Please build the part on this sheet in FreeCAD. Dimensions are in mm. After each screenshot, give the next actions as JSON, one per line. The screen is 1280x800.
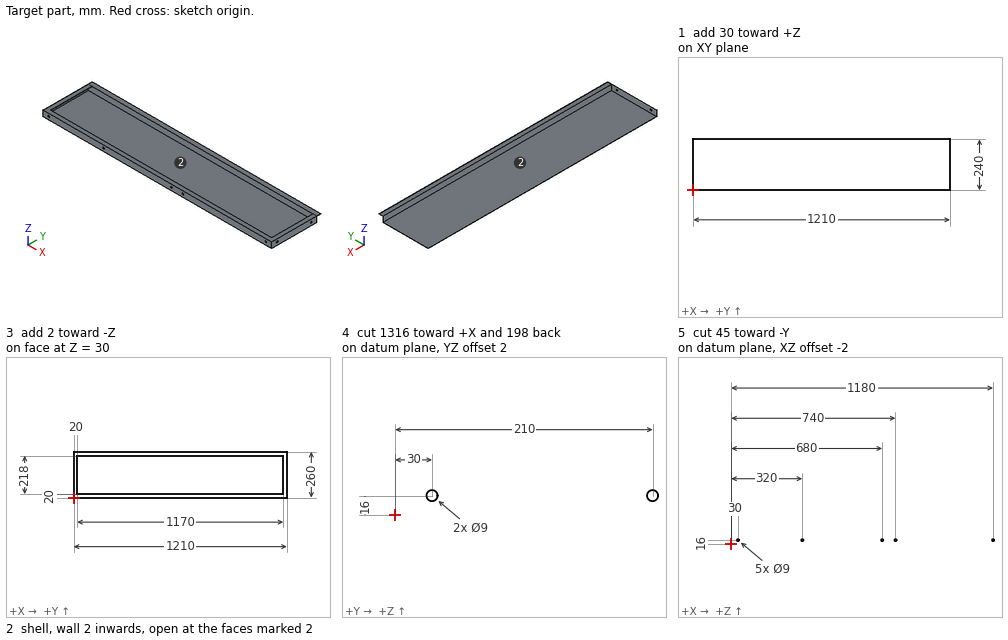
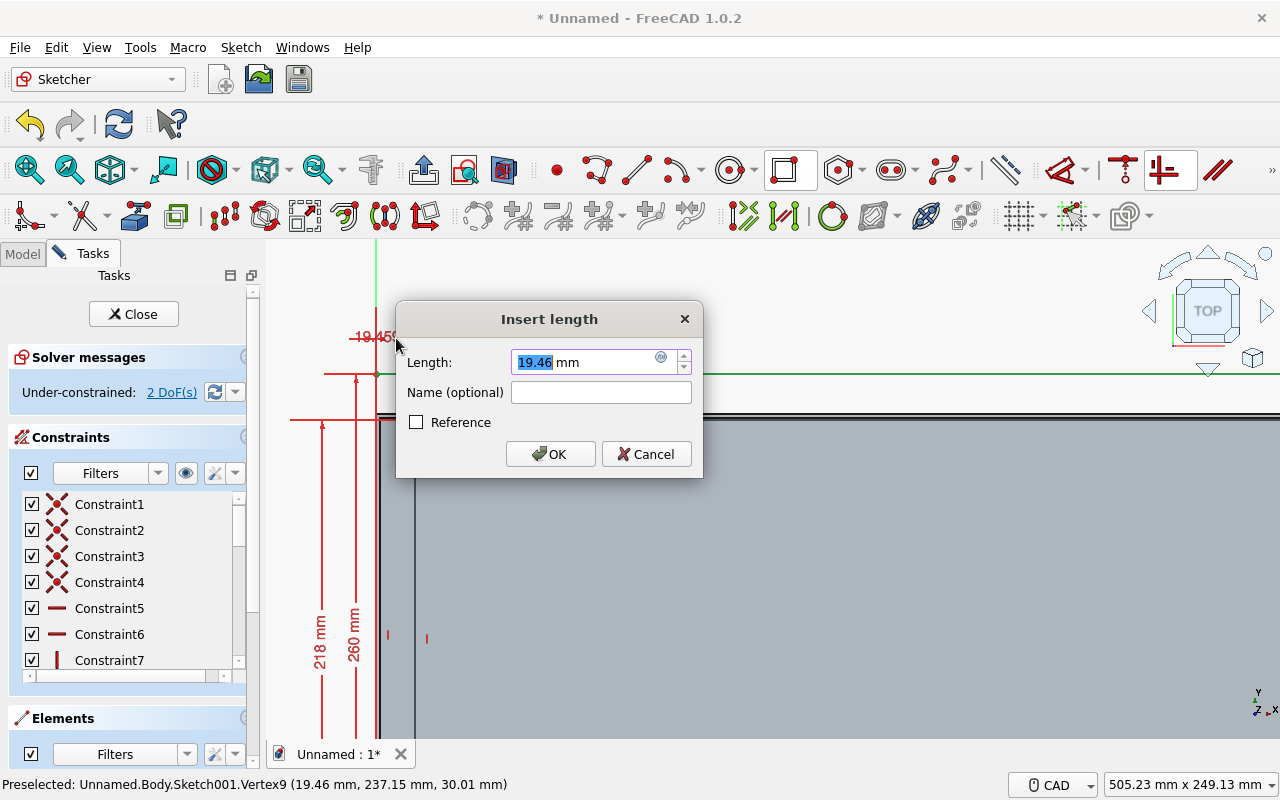
{"action": "type", "text": "20"}
{"action": "key", "text": "Return"}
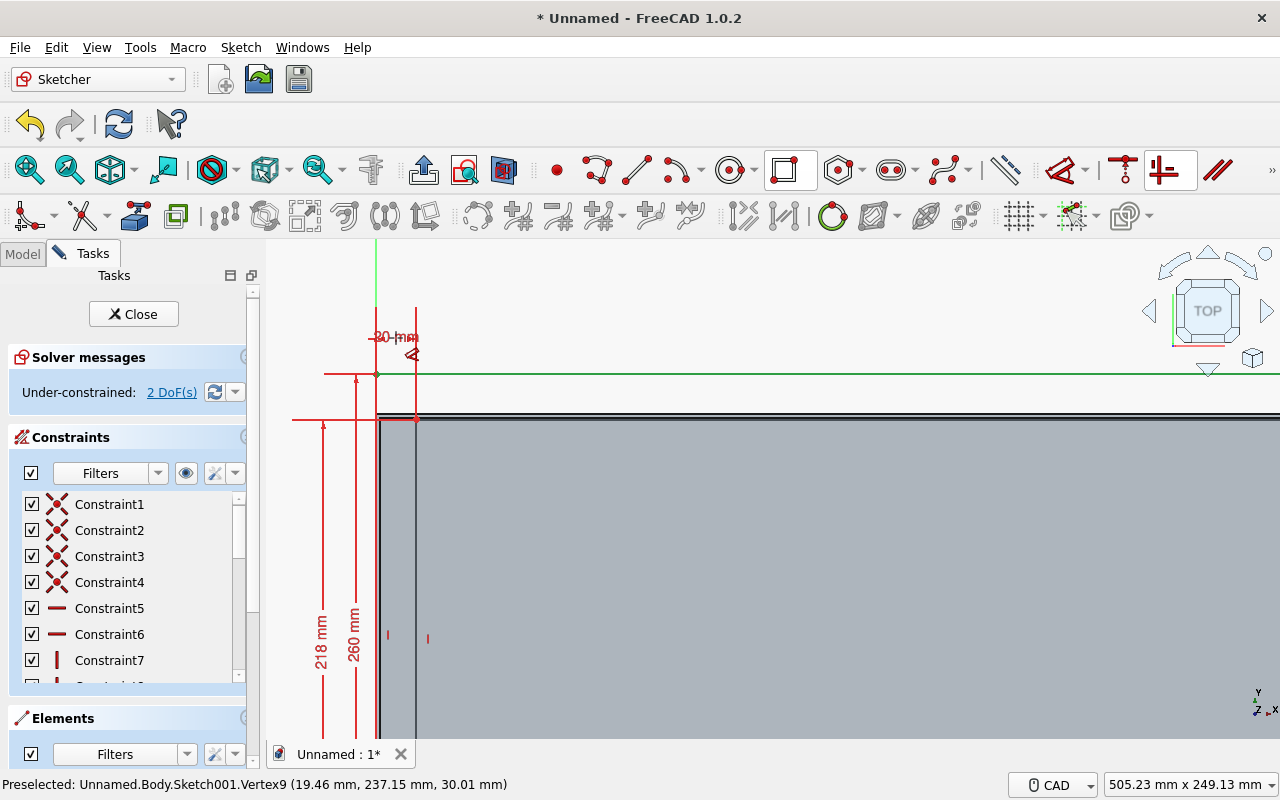
{"action": "scroll", "coordinate": [415, 441], "scroll_direction": "down", "scroll_amount": 7}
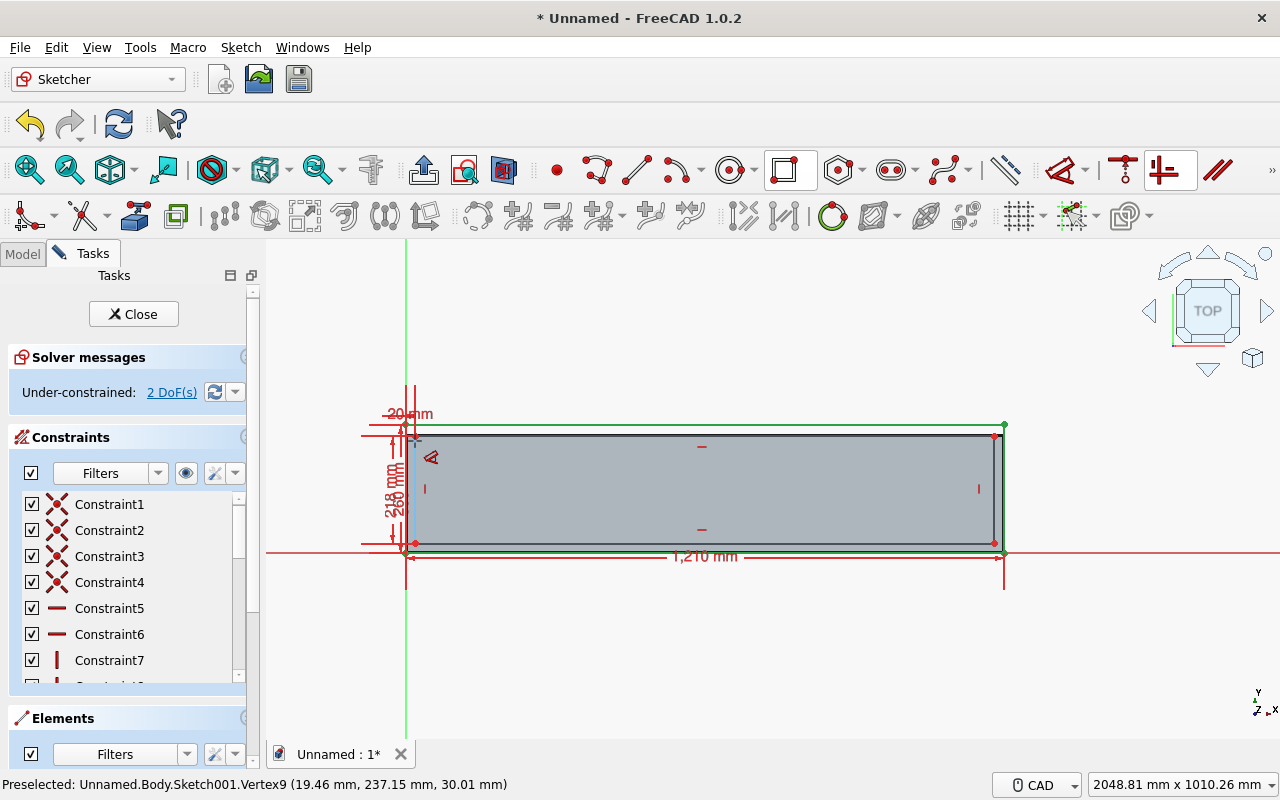
{"action": "scroll", "coordinate": [415, 544], "scroll_direction": "up", "scroll_amount": 7}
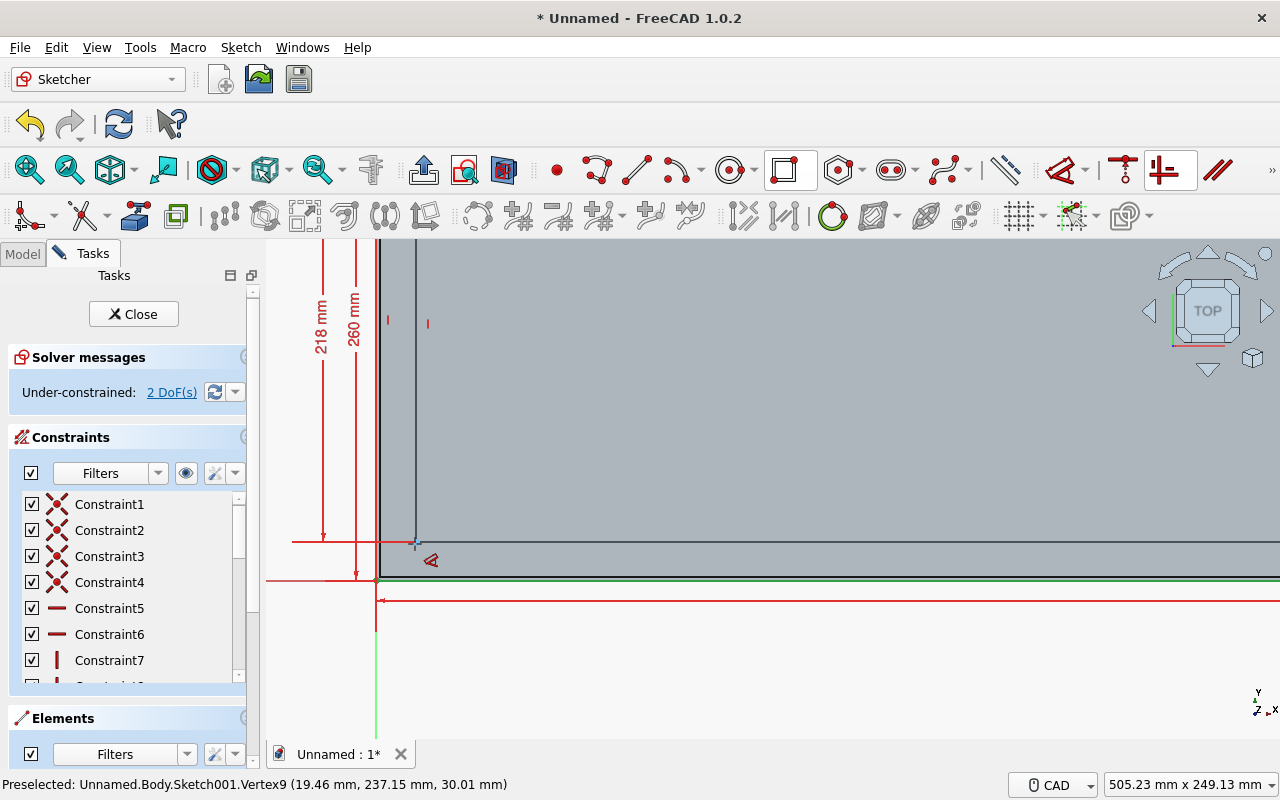
{"action": "left_click", "coordinate": [416, 542]}
{"action": "left_click", "coordinate": [342, 561]}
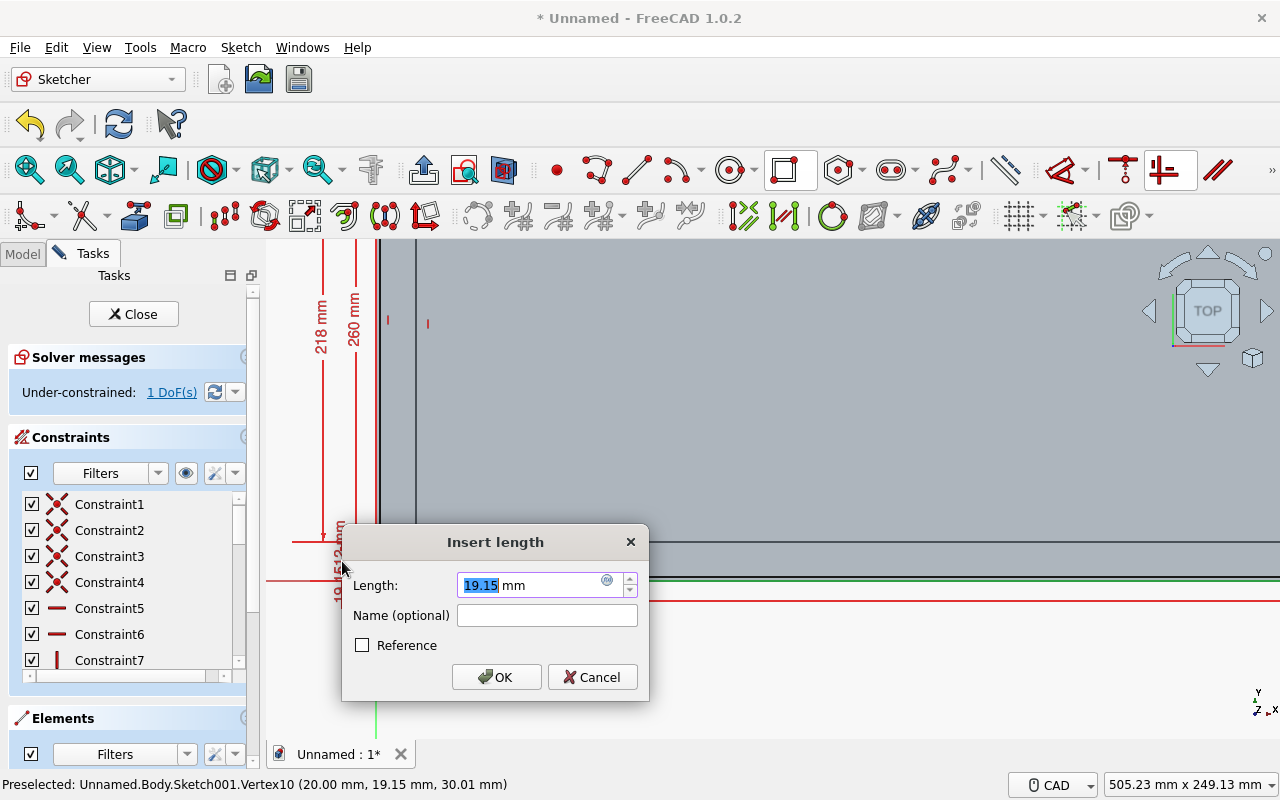
{"action": "type", "text": "20"}
{"action": "key", "text": "Return"}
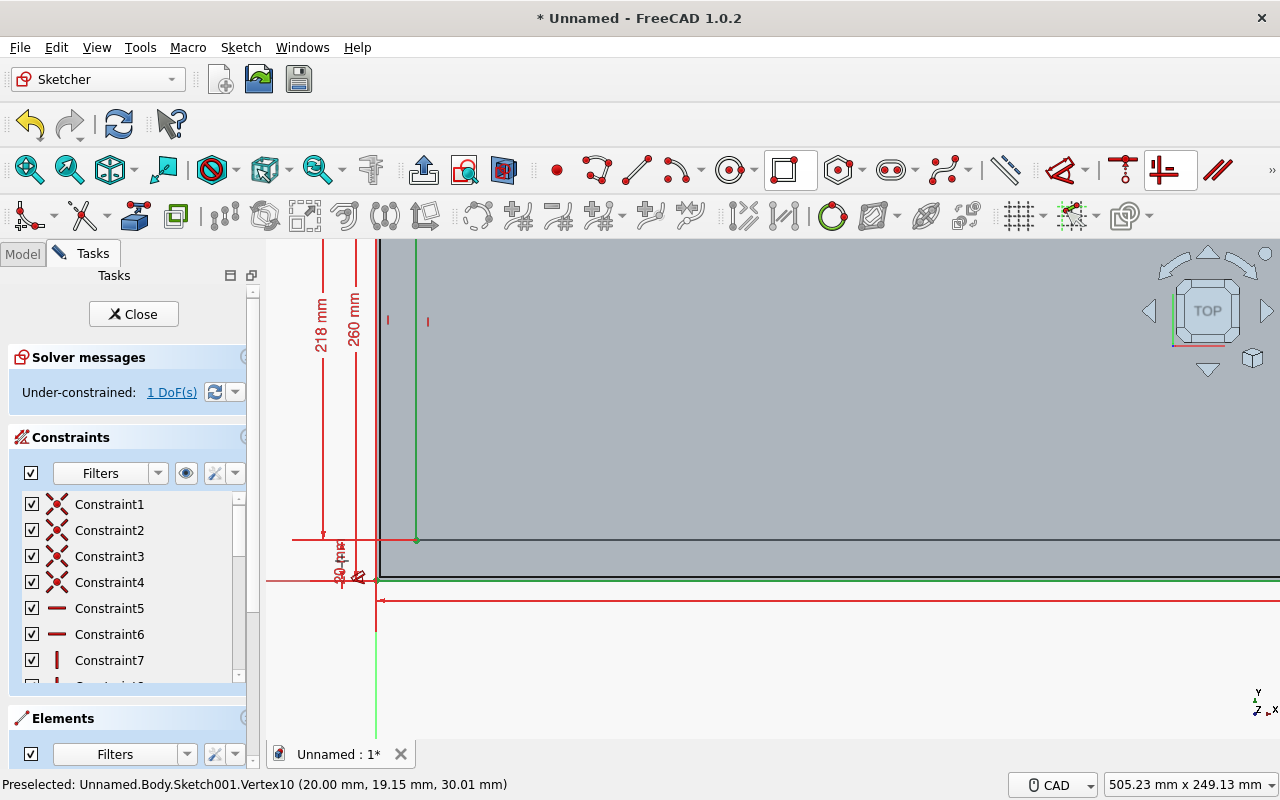
{"action": "left_click", "coordinate": [886, 540]}
{"action": "left_click", "coordinate": [766, 506]}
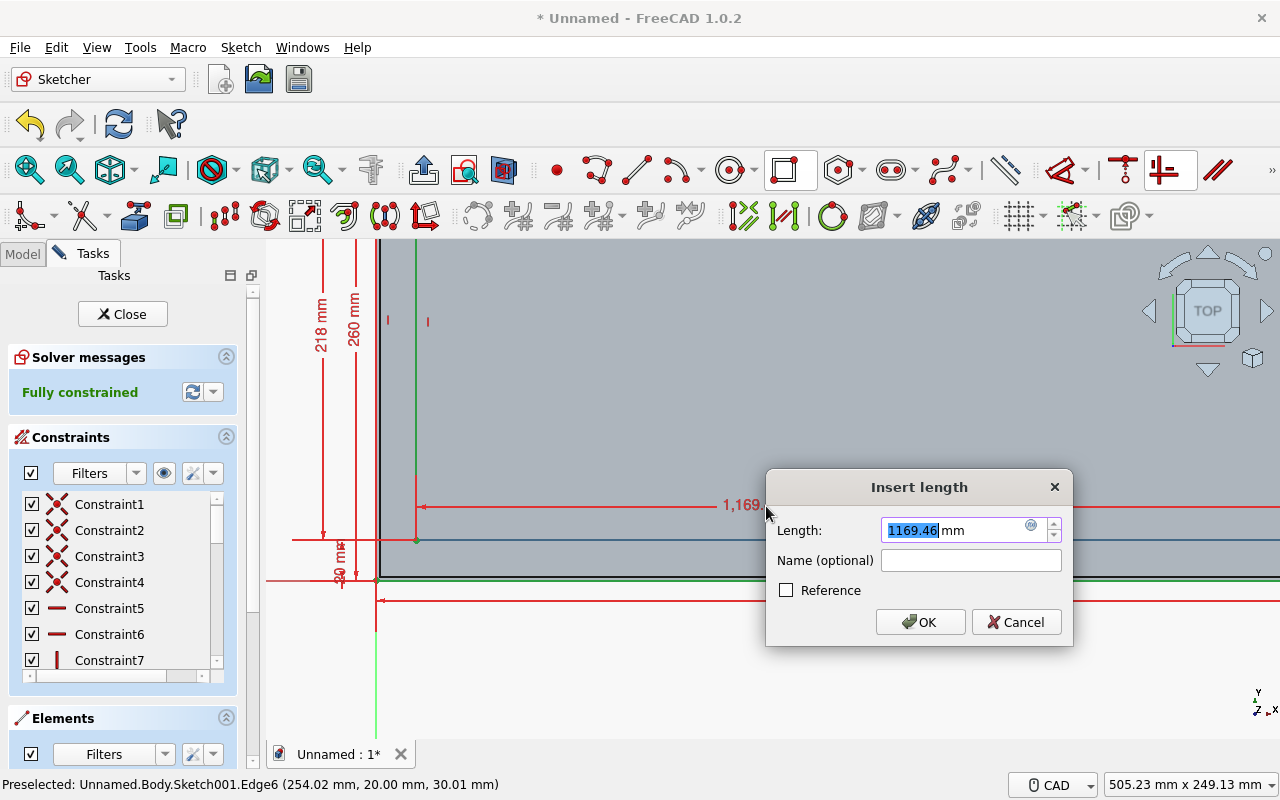
{"action": "type", "text": "1170"}
{"action": "key", "text": "Return"}
{"action": "key", "text": "Escape"}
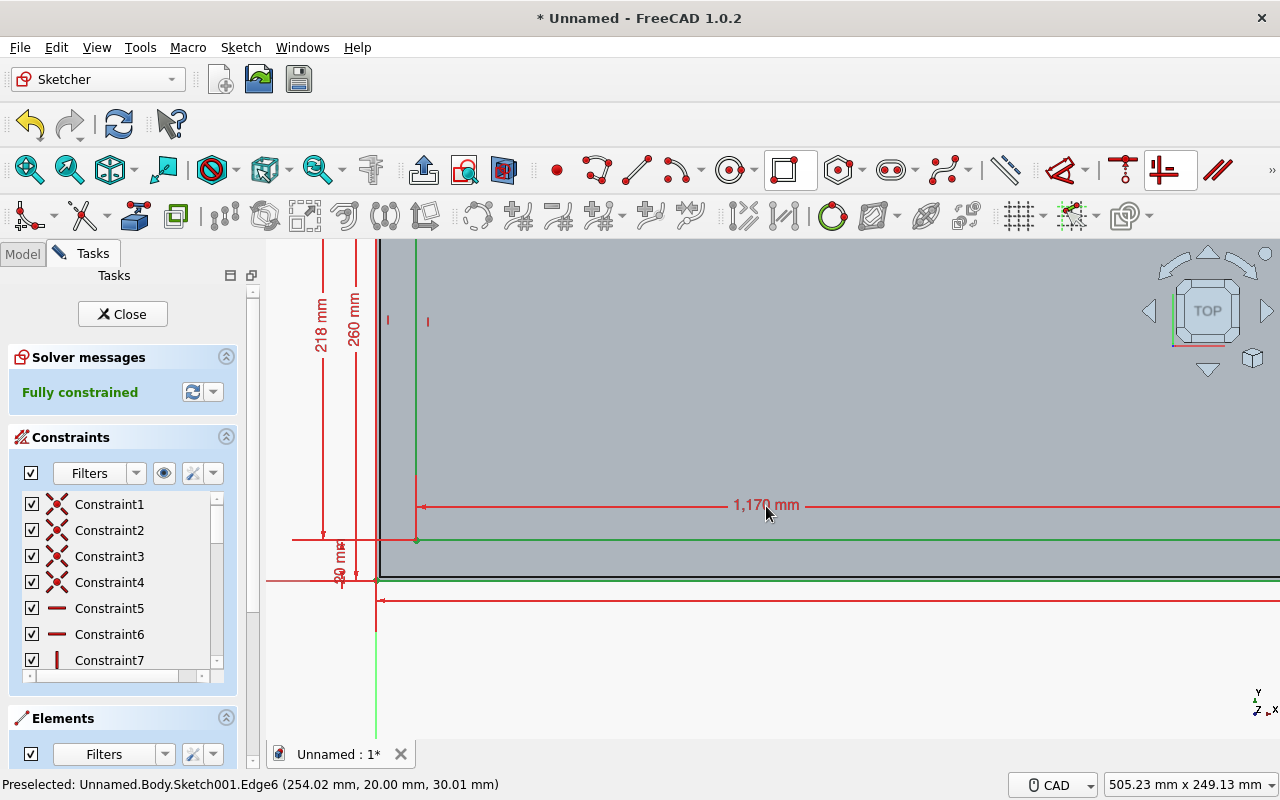
{"action": "left_click", "coordinate": [123, 314]}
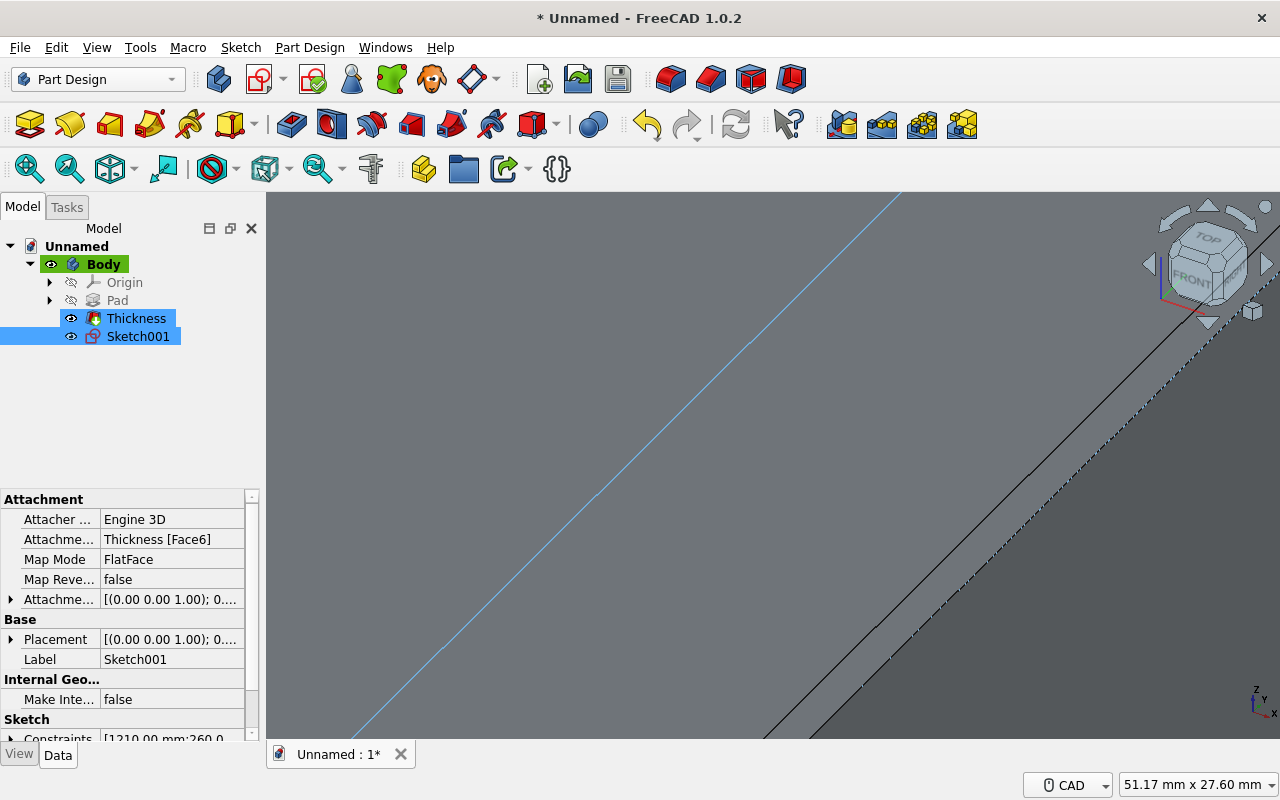
{"action": "left_click", "coordinate": [30, 124]}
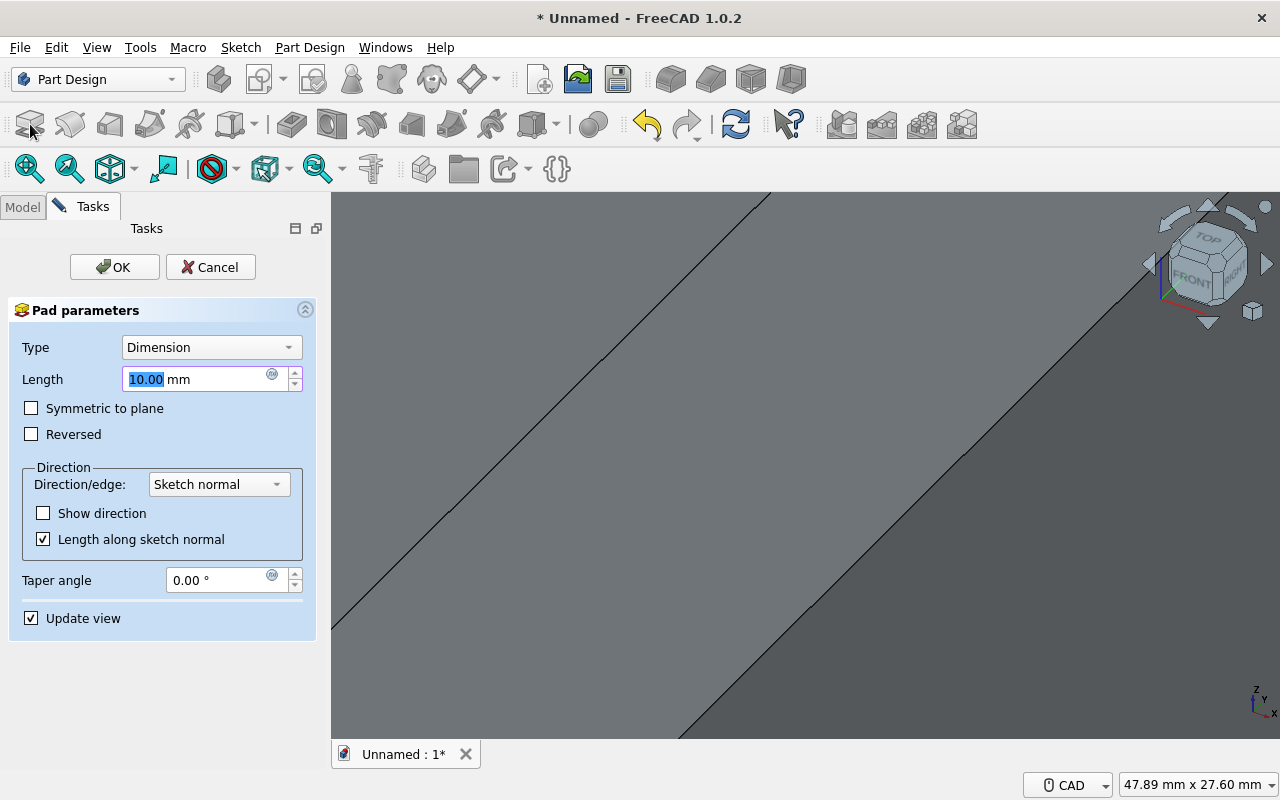
{"action": "type", "text": "2"}
{"action": "key", "text": "Tab"}